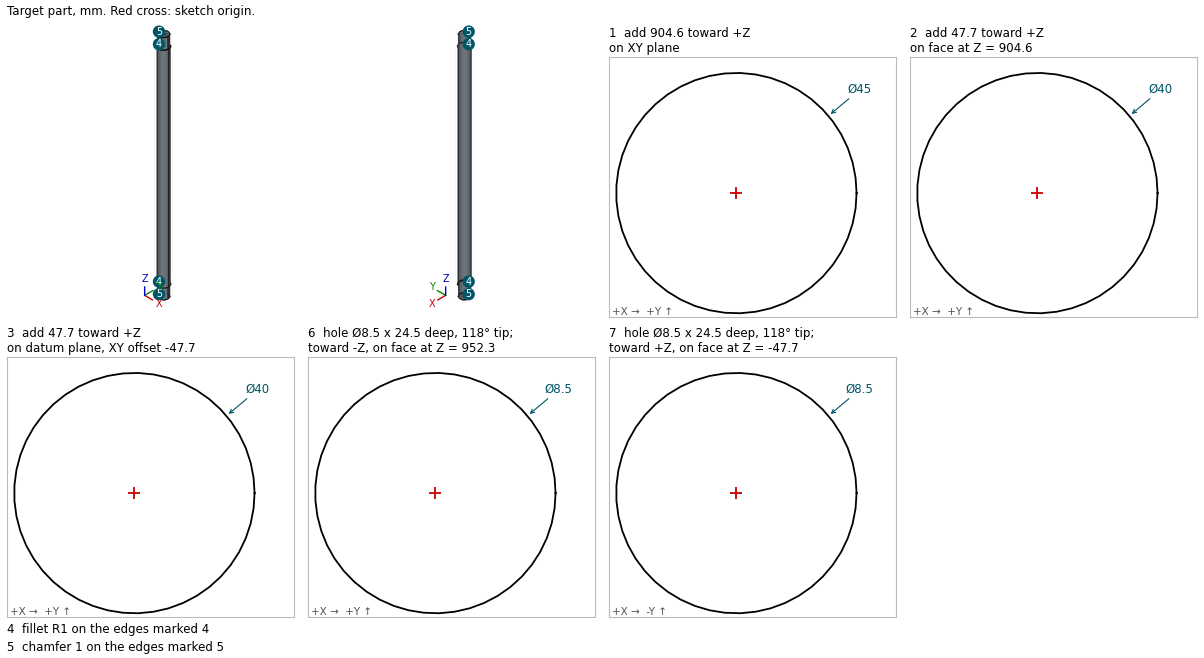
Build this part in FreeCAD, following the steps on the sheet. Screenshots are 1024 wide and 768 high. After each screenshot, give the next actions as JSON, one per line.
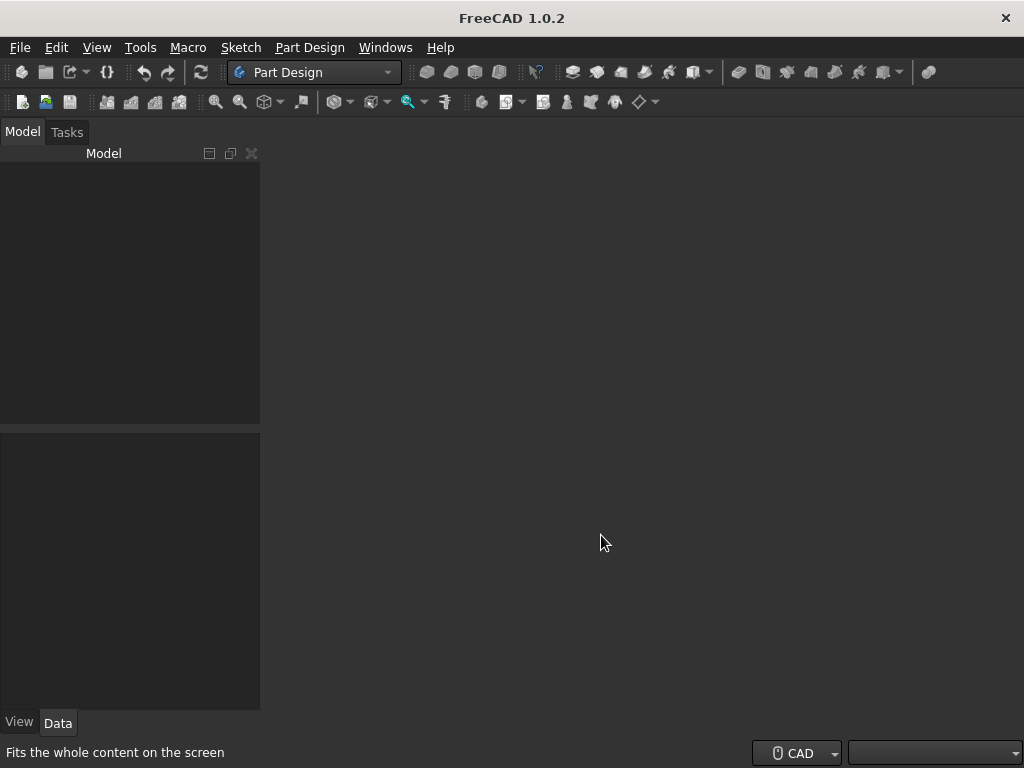
{"action": "left_click", "coordinate": [22, 102]}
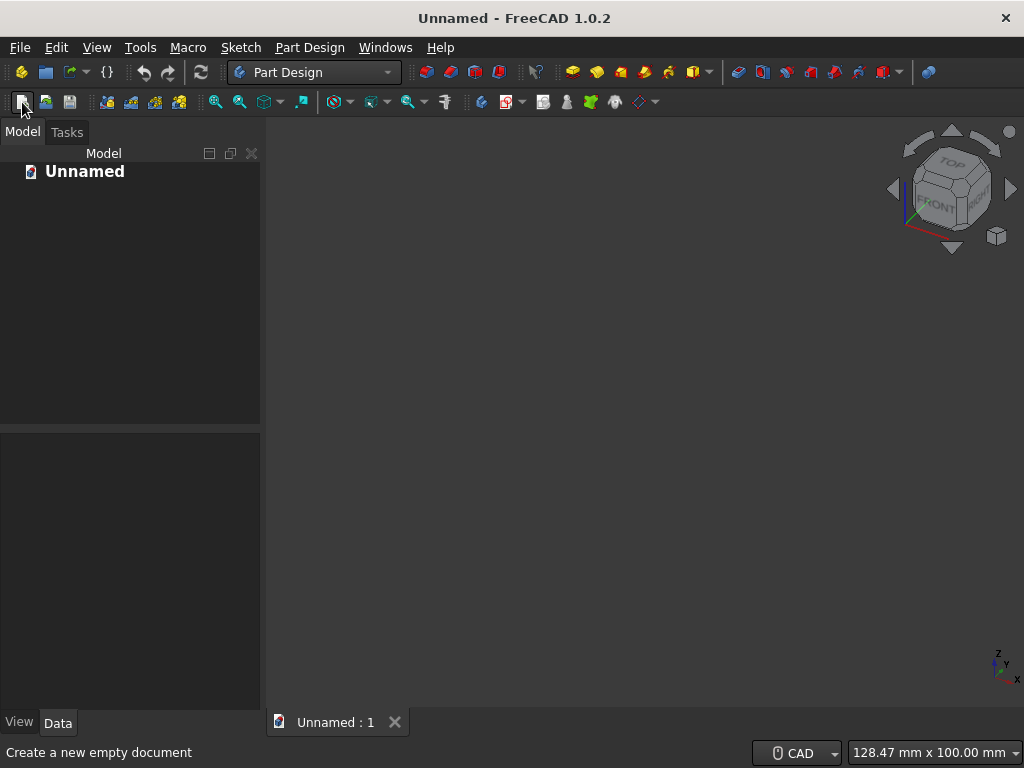
{"action": "left_click", "coordinate": [506, 102]}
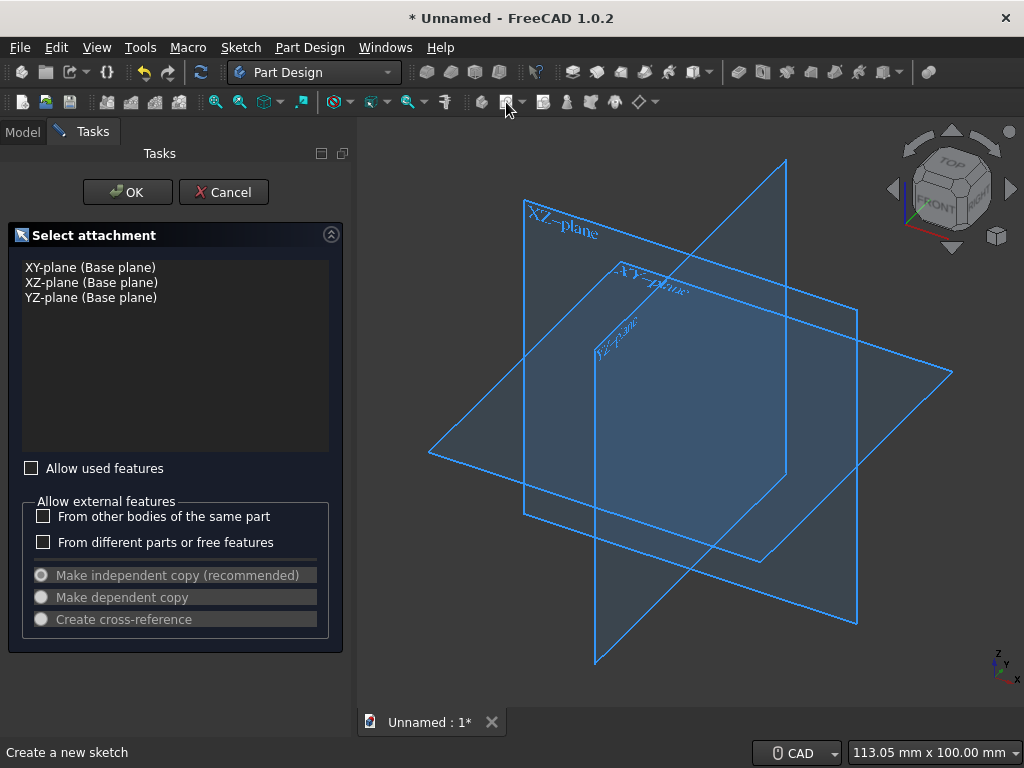
{"action": "left_click", "coordinate": [82, 268]}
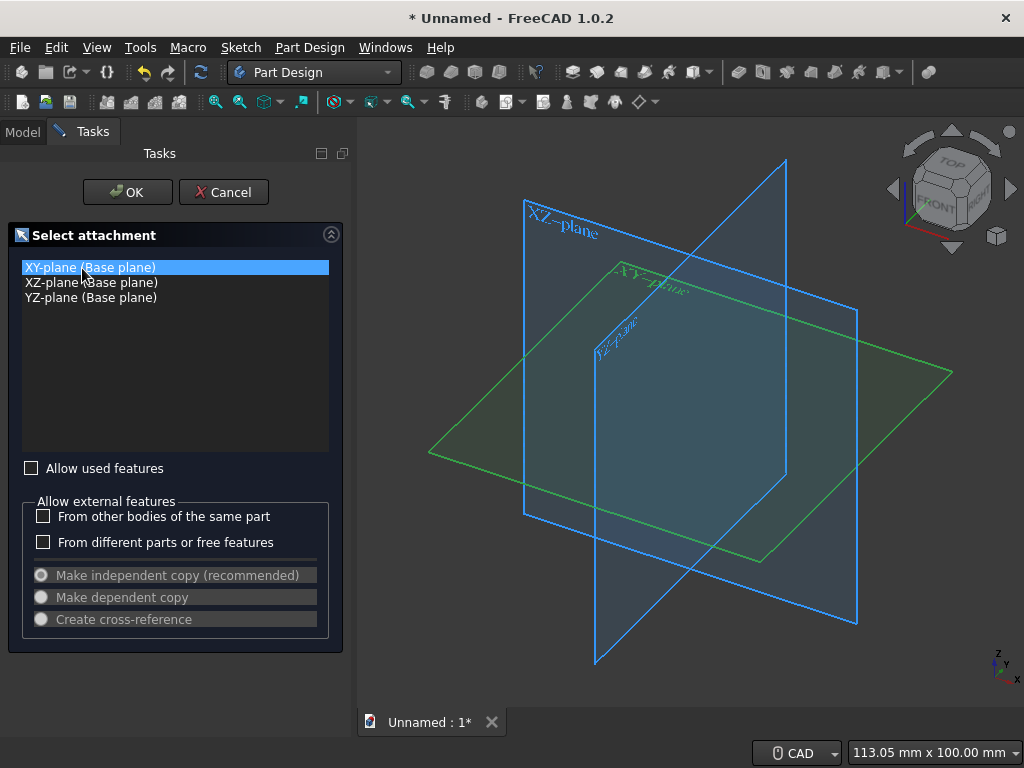
{"action": "left_click", "coordinate": [128, 192]}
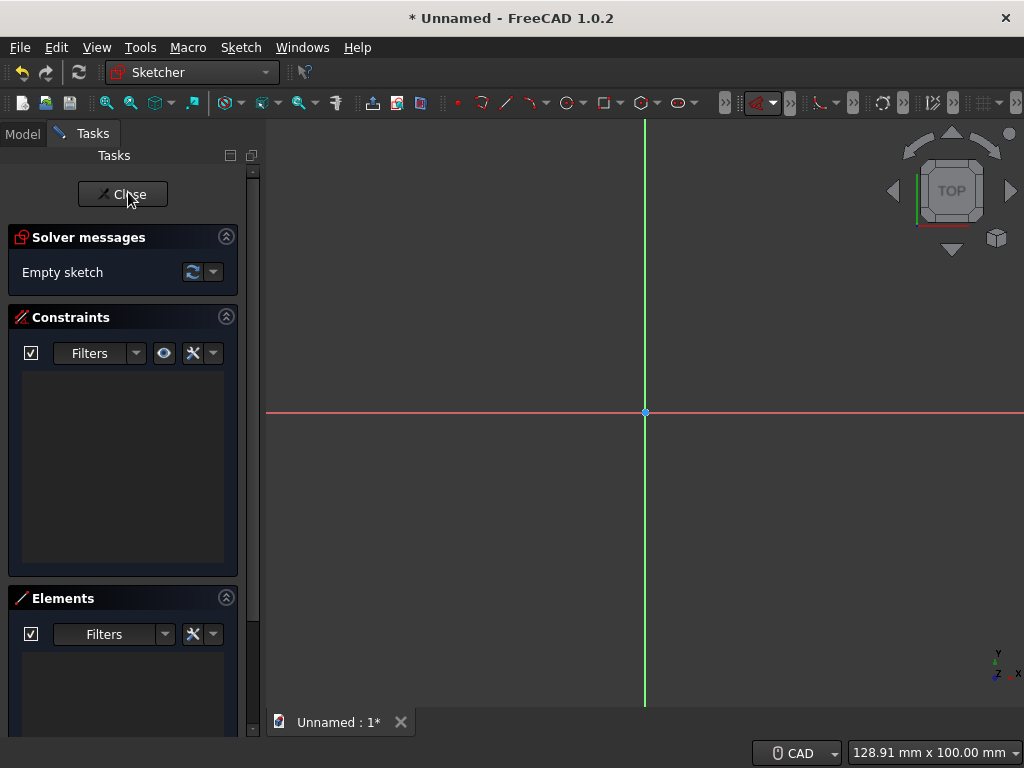
{"action": "scroll", "coordinate": [784, 413], "scroll_direction": "up", "scroll_amount": 2}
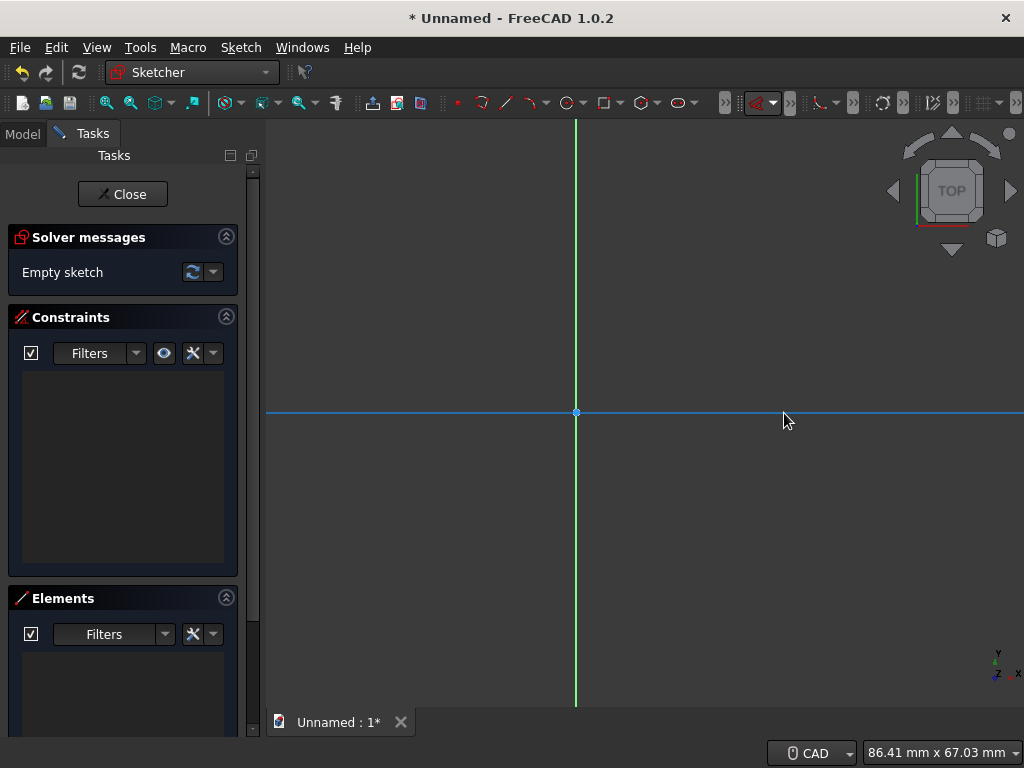
{"action": "left_click", "coordinate": [568, 104]}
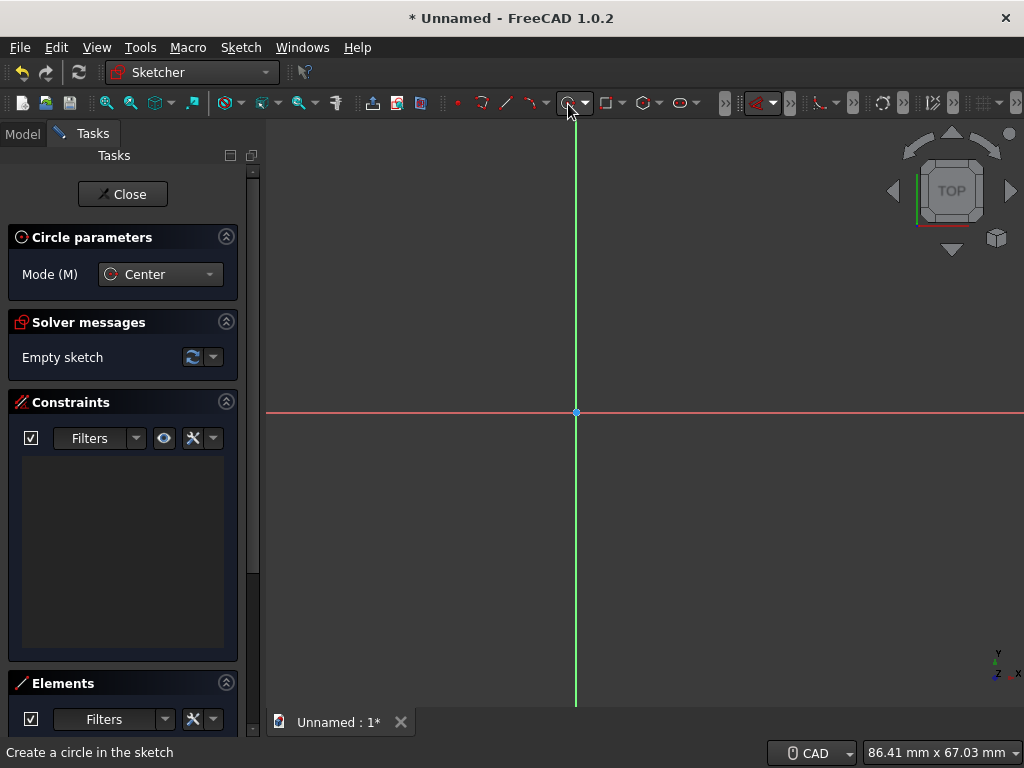
{"action": "left_click", "coordinate": [576, 413]}
{"action": "mouse_move", "coordinate": [716, 273]}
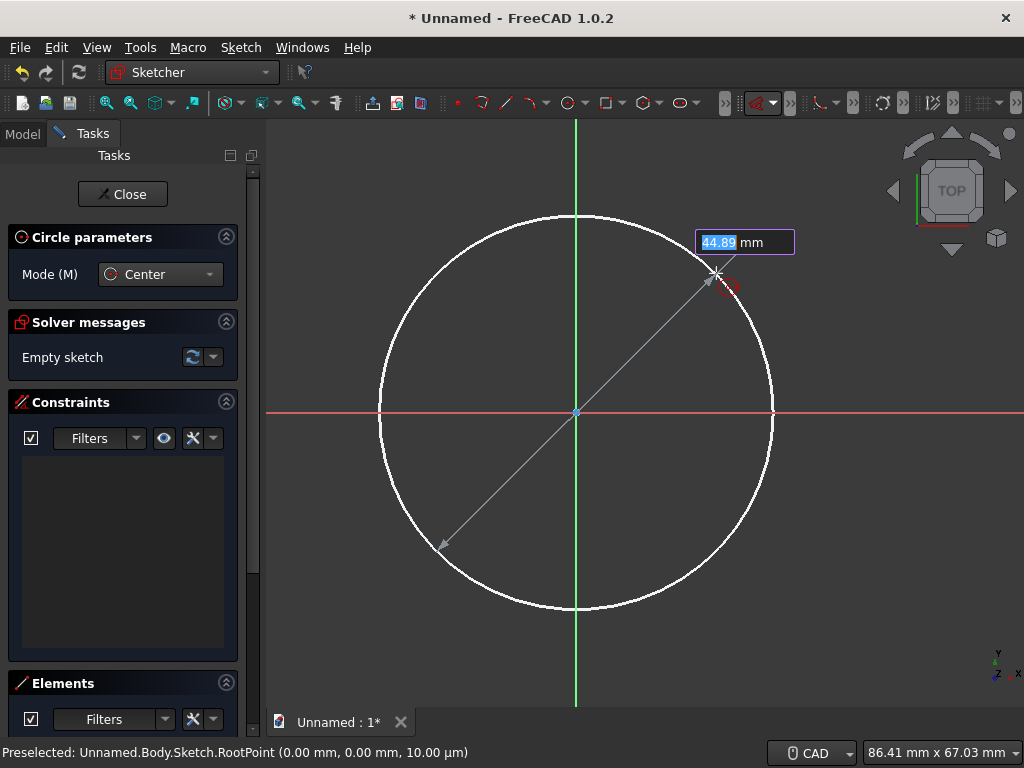
{"action": "type", "text": "45"}
{"action": "key", "text": "Return"}
{"action": "key", "text": "Escape"}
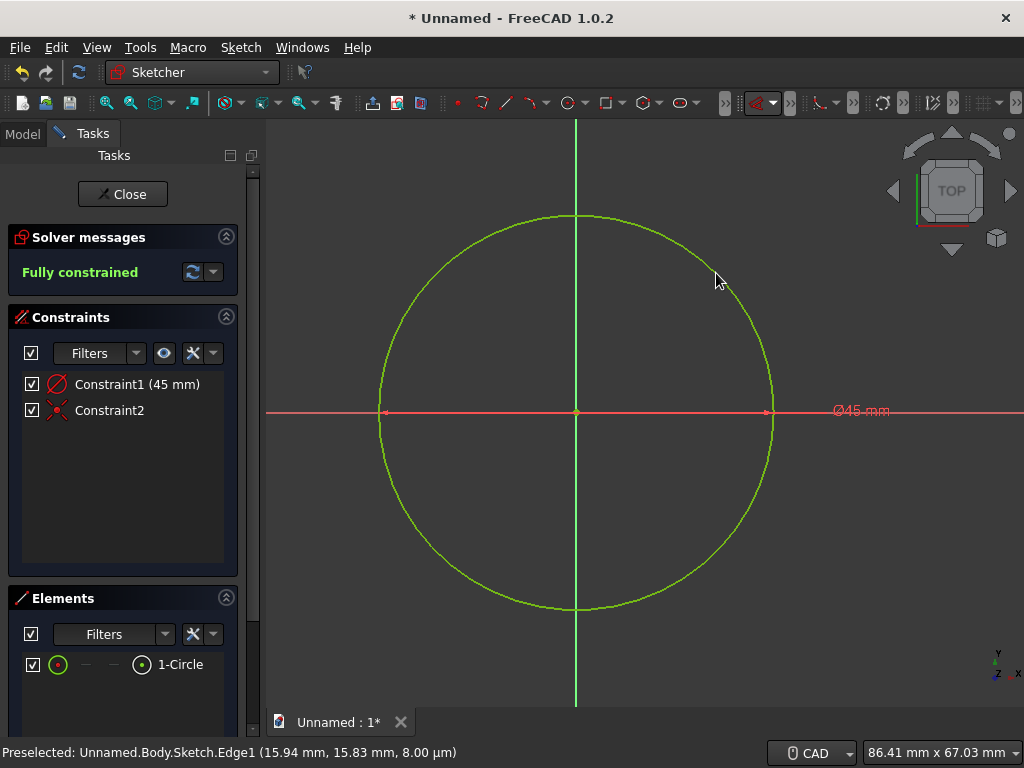
{"action": "left_click", "coordinate": [123, 194]}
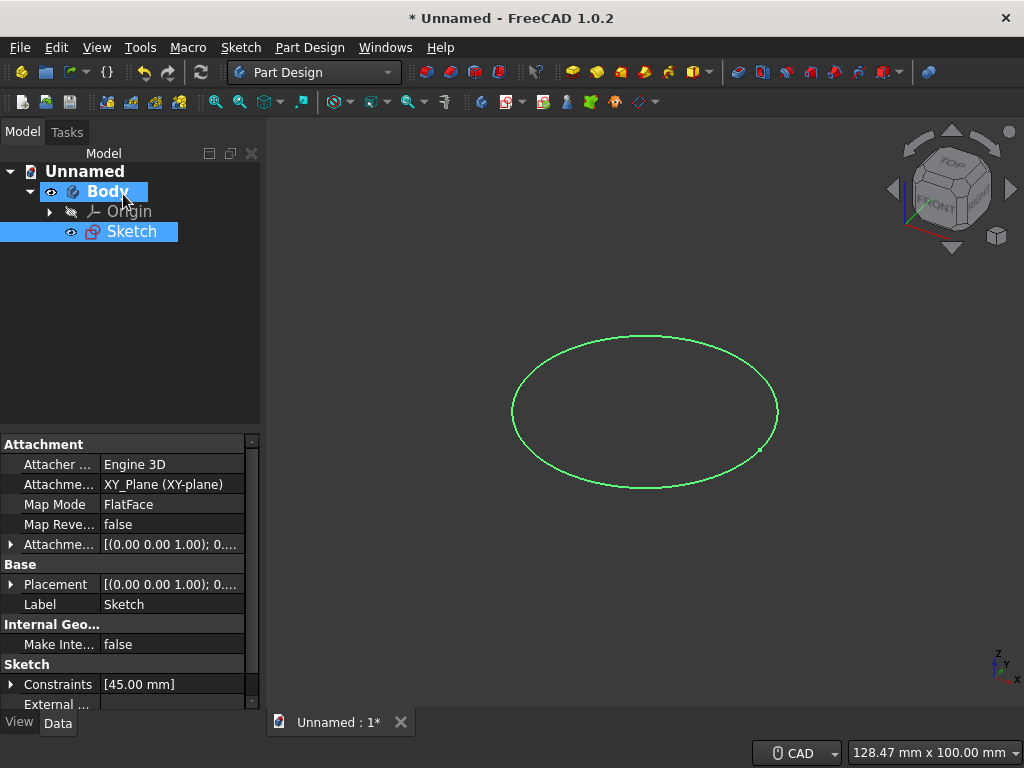
{"action": "left_click", "coordinate": [574, 72]}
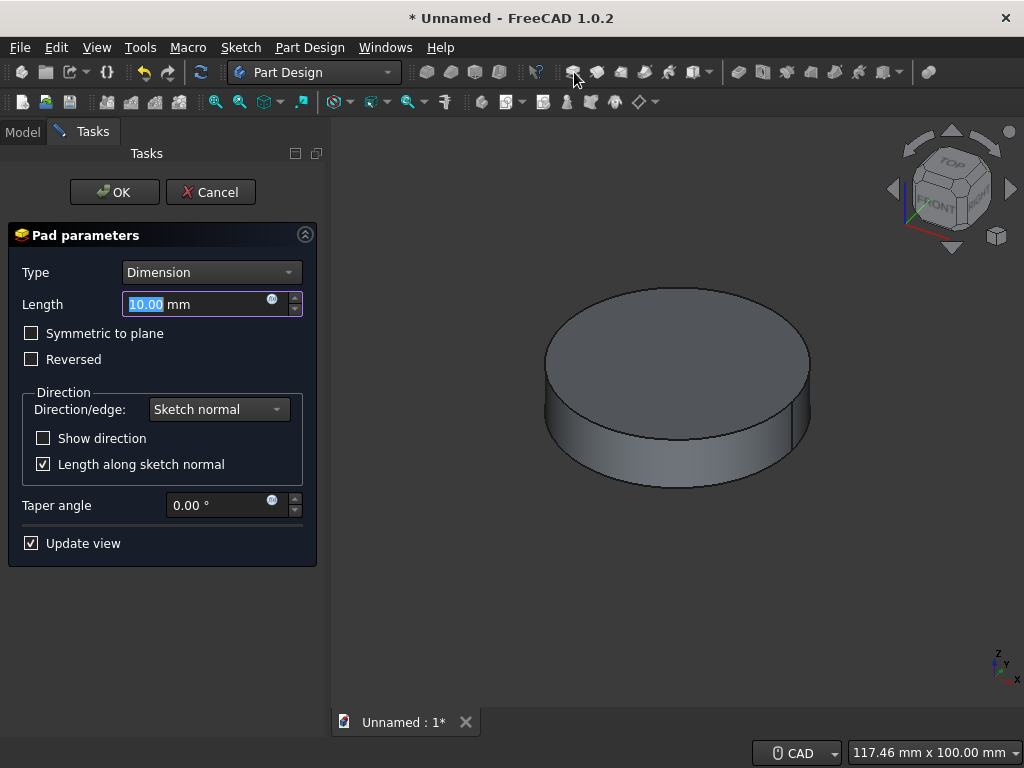
{"action": "type", "text": "904.6"}
{"action": "key", "text": "Tab"}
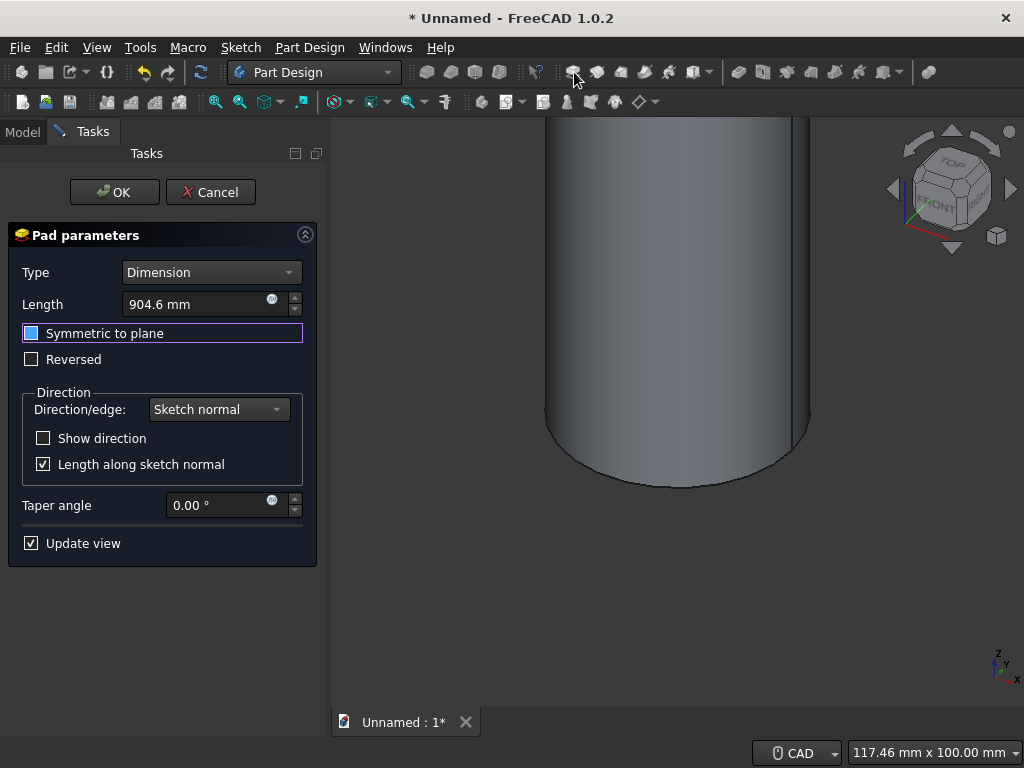
{"action": "left_click", "coordinate": [115, 192]}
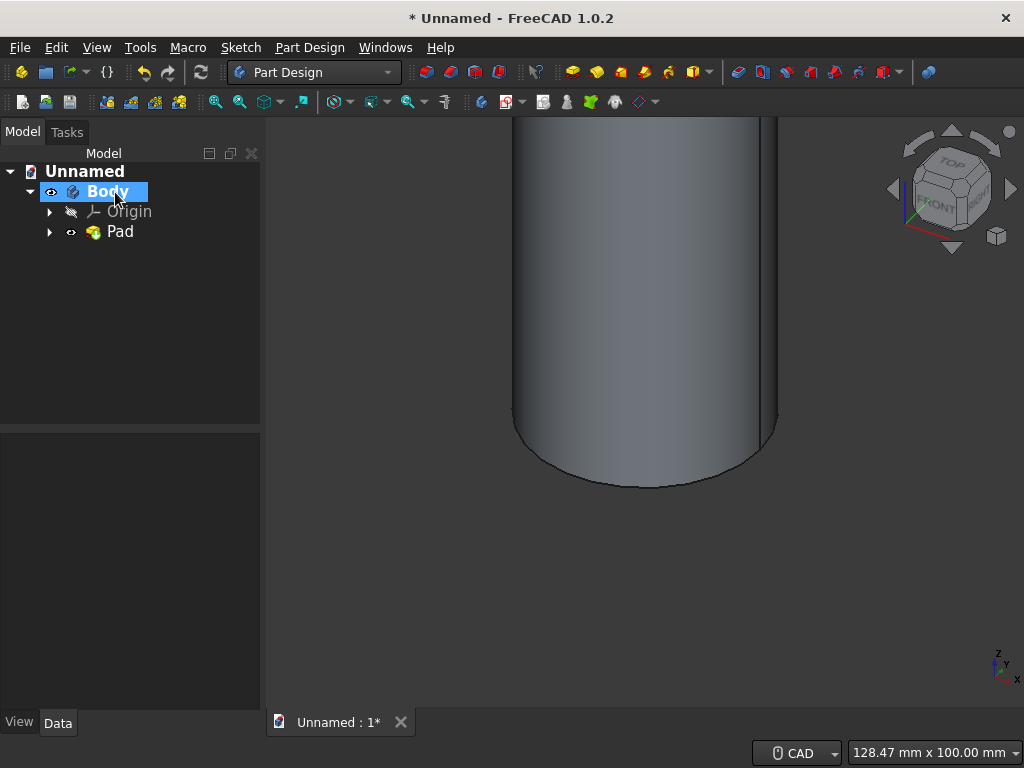
{"action": "left_click", "coordinate": [216, 102]}